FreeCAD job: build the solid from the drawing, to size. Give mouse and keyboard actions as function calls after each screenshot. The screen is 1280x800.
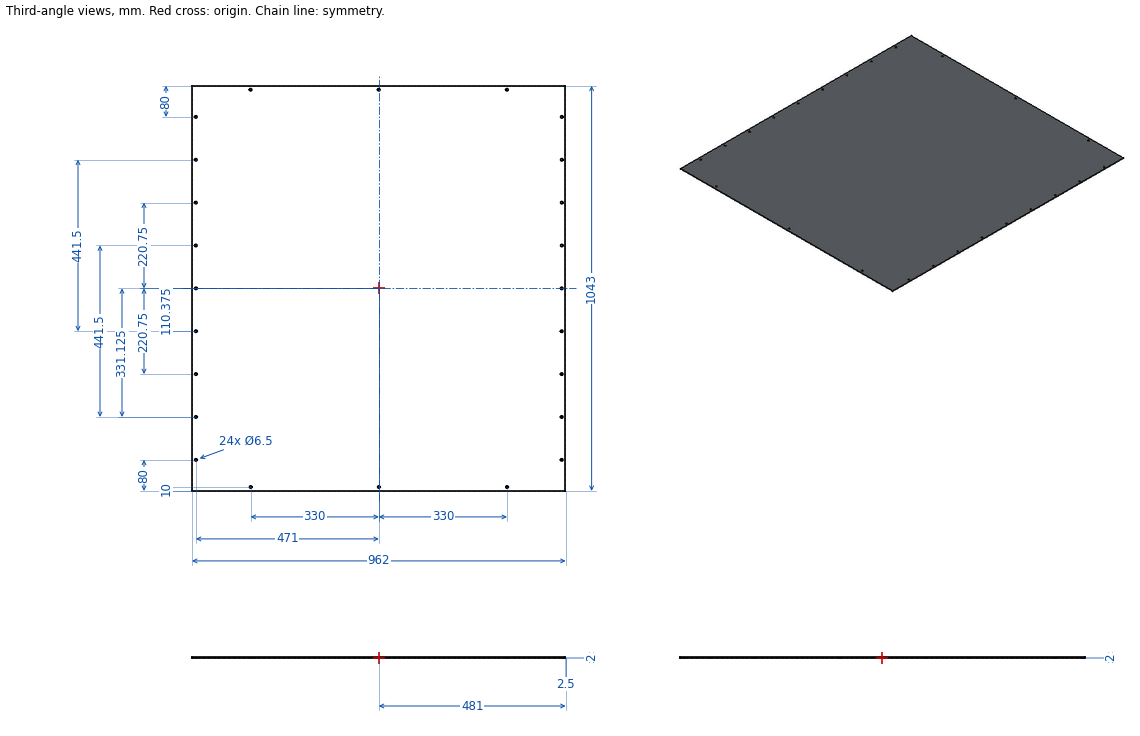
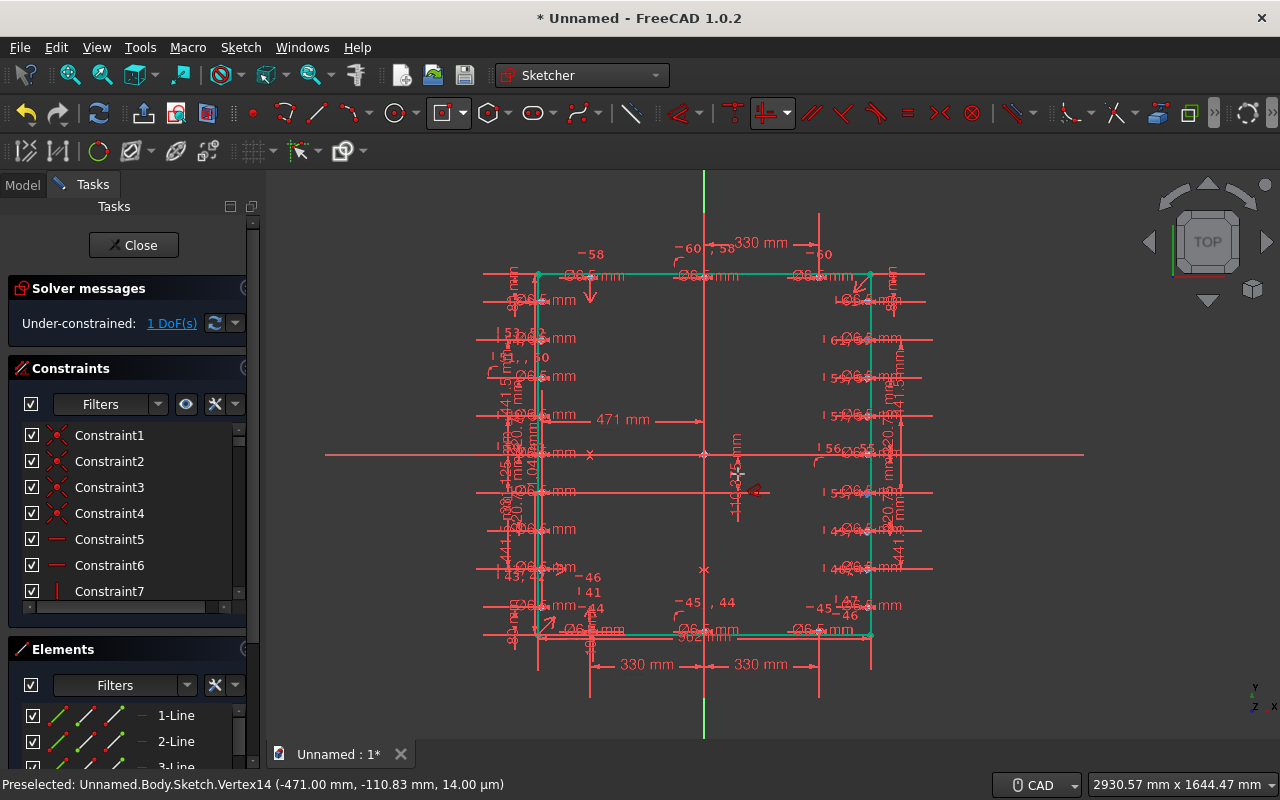
click(867, 493)
click(646, 474)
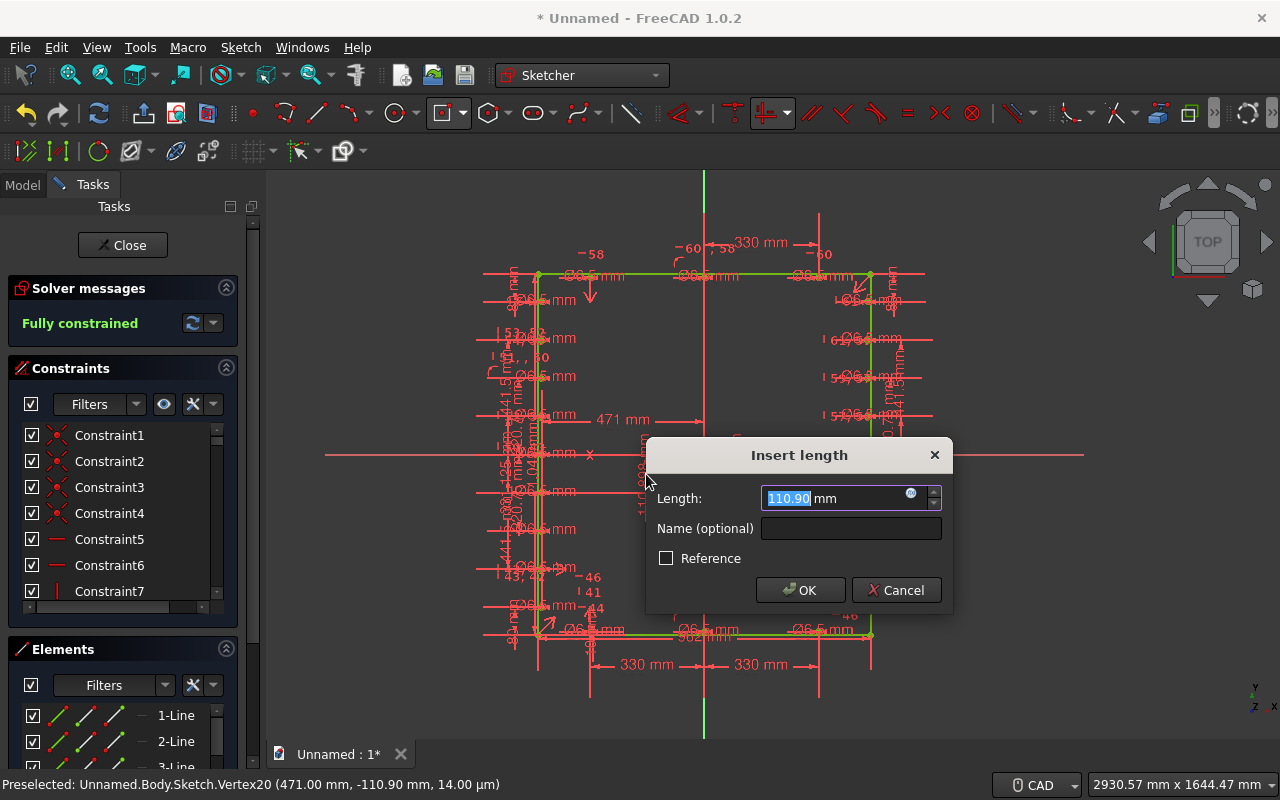
text(110.375)
key(Return)
key(Escape)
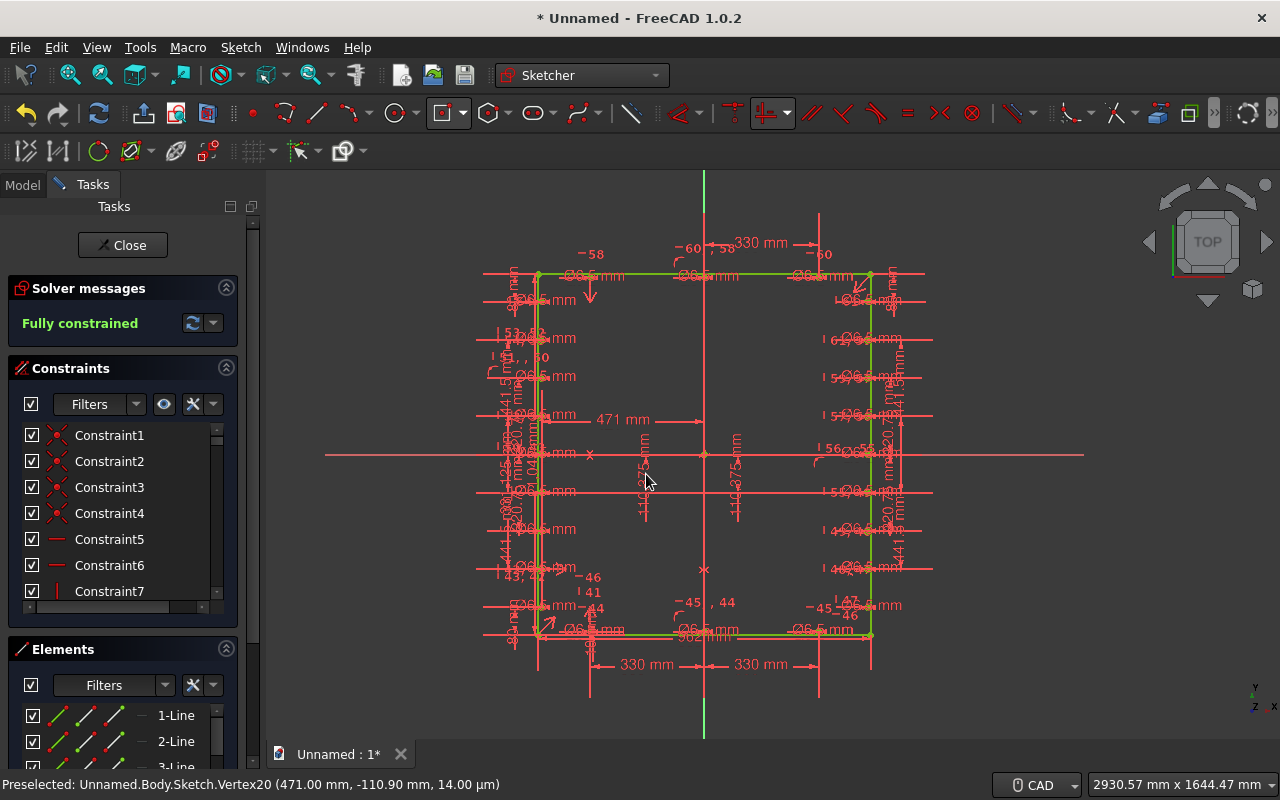
click(123, 245)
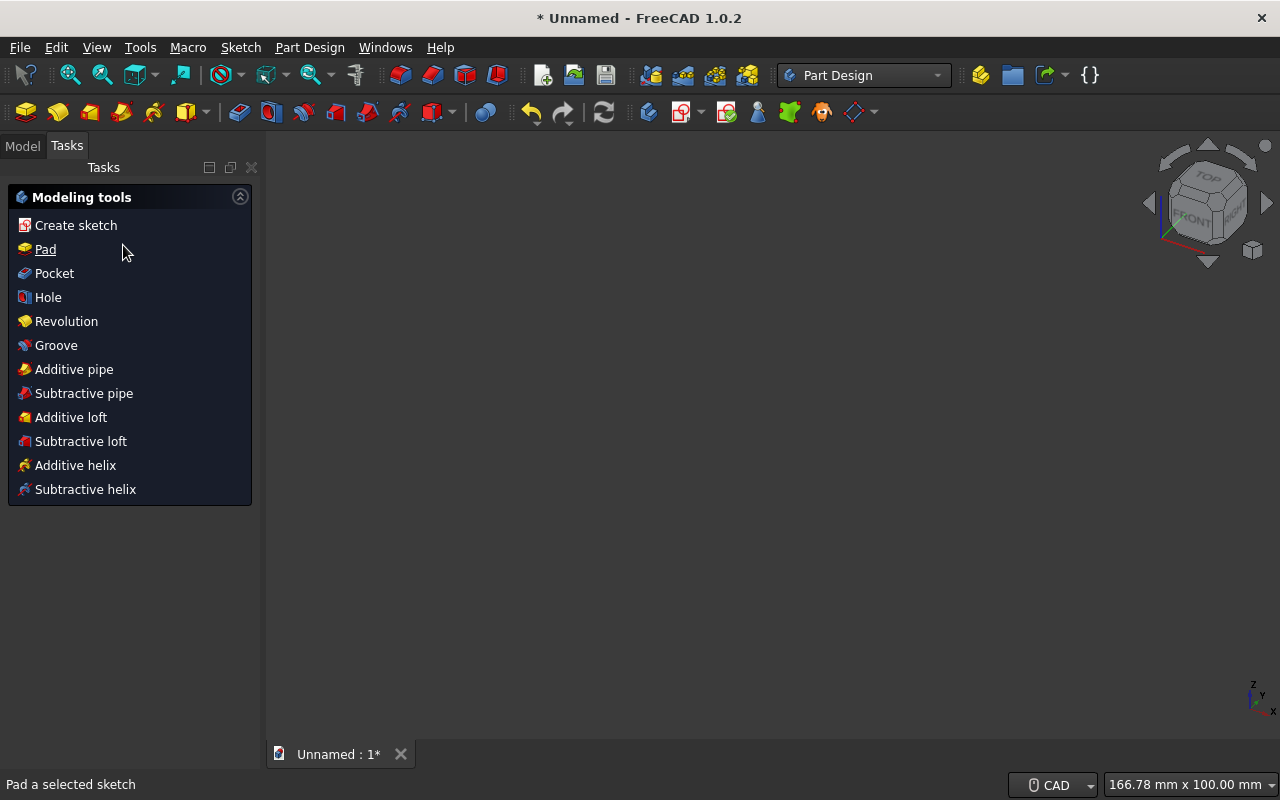
click(26, 112)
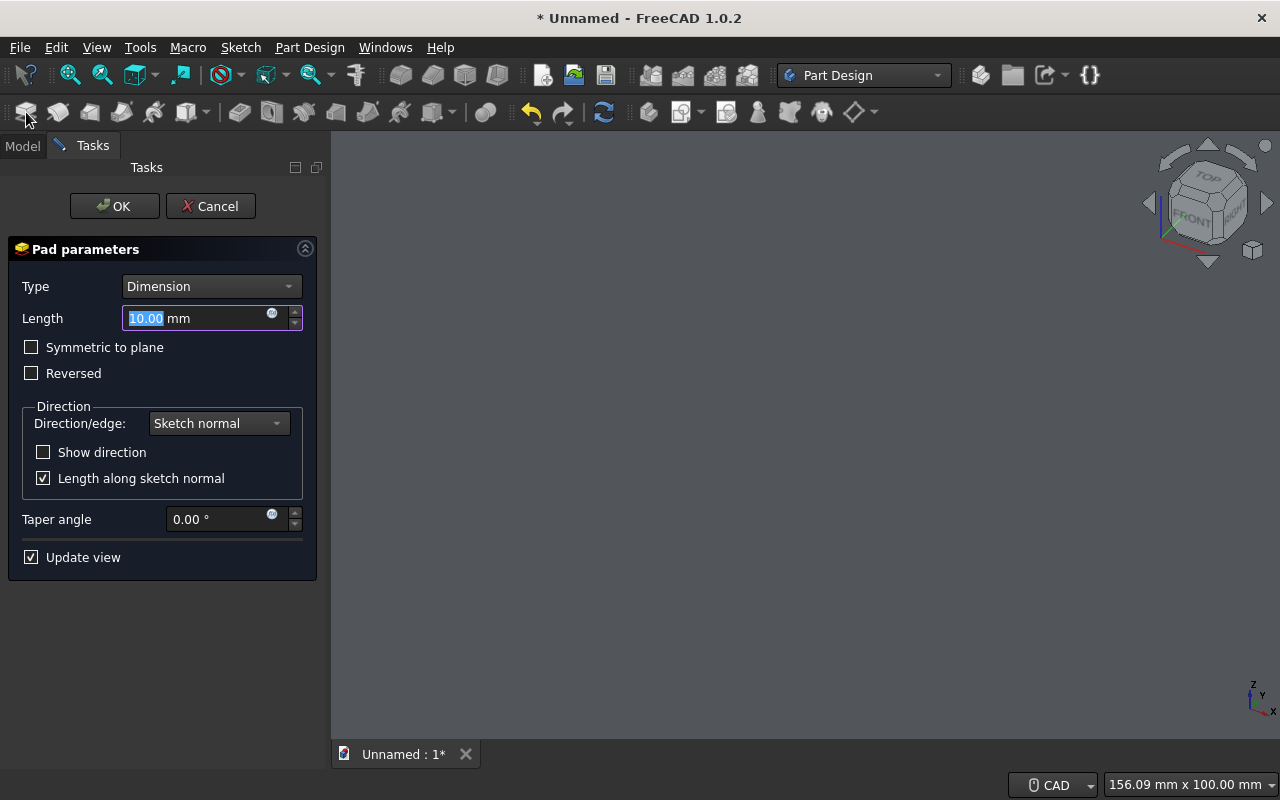
text(2)
key(Tab)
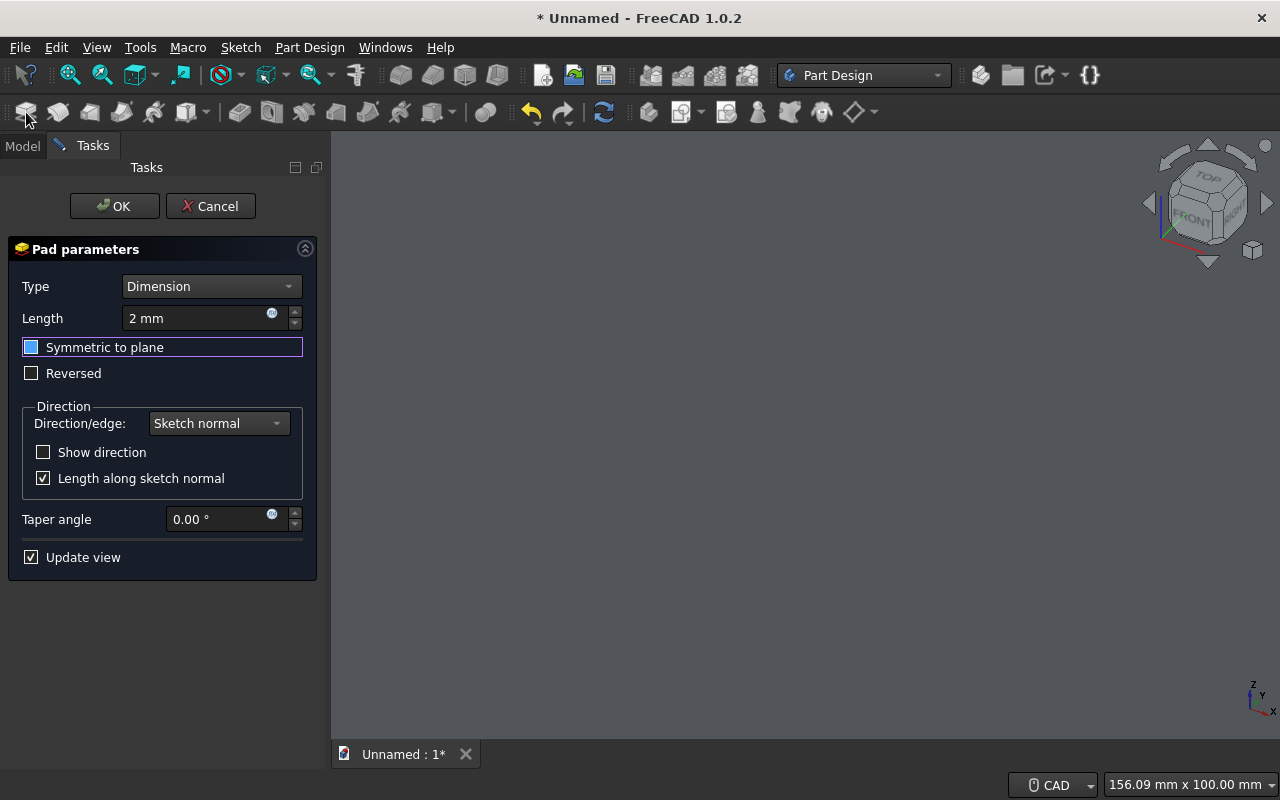
click(115, 206)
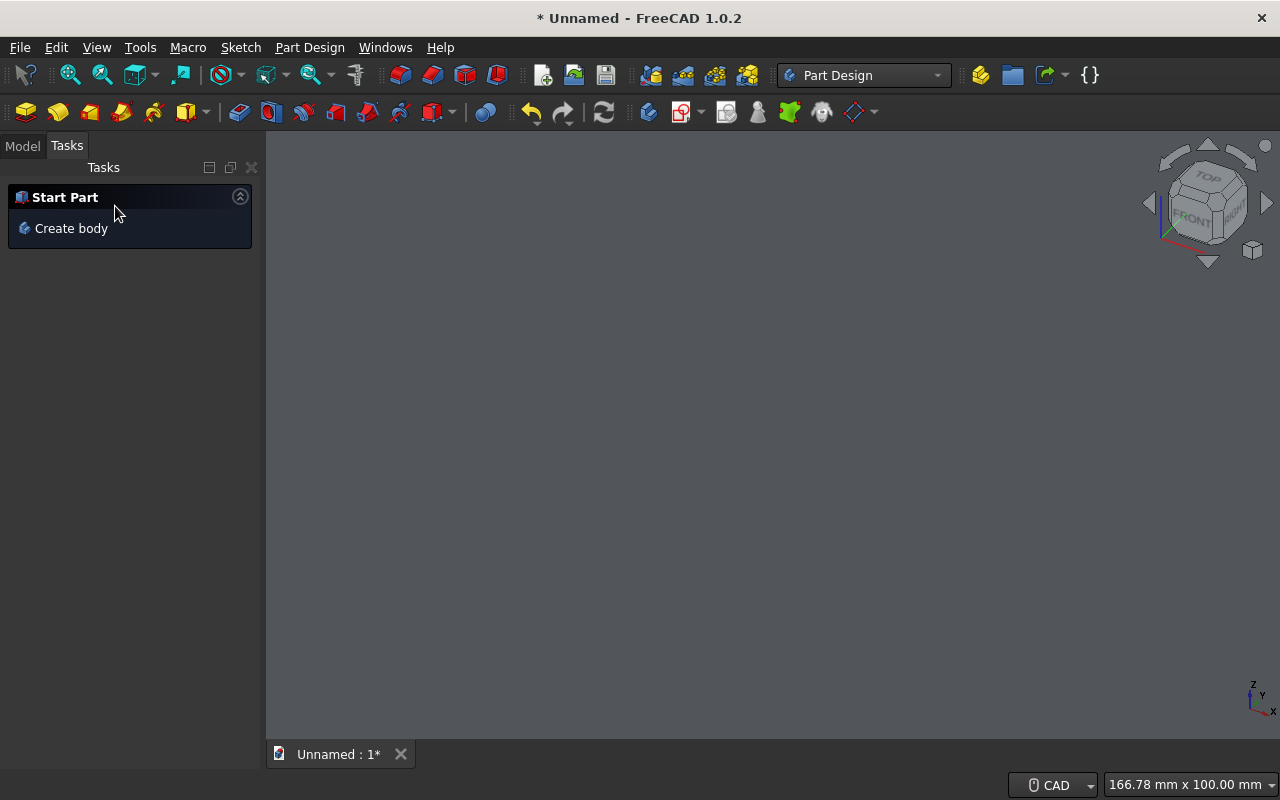
click(72, 76)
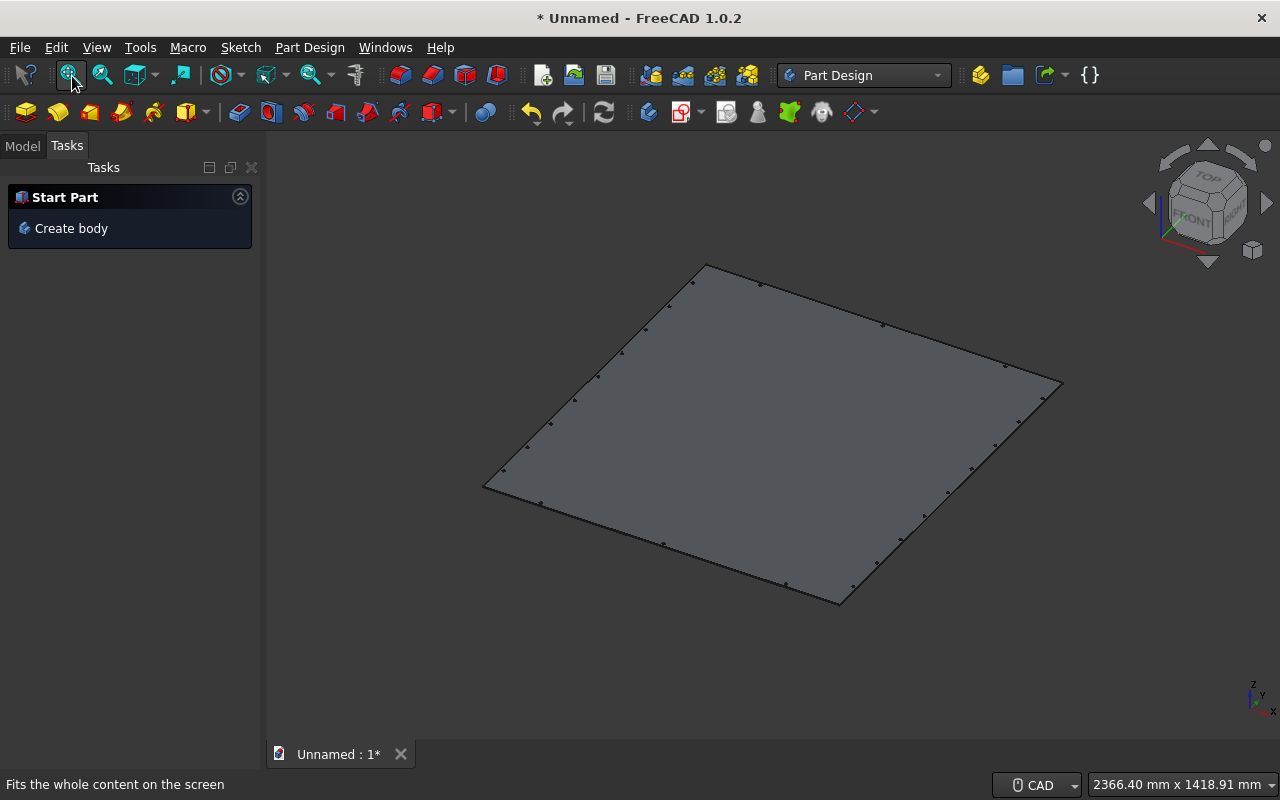
scroll(814, 596, up, 15)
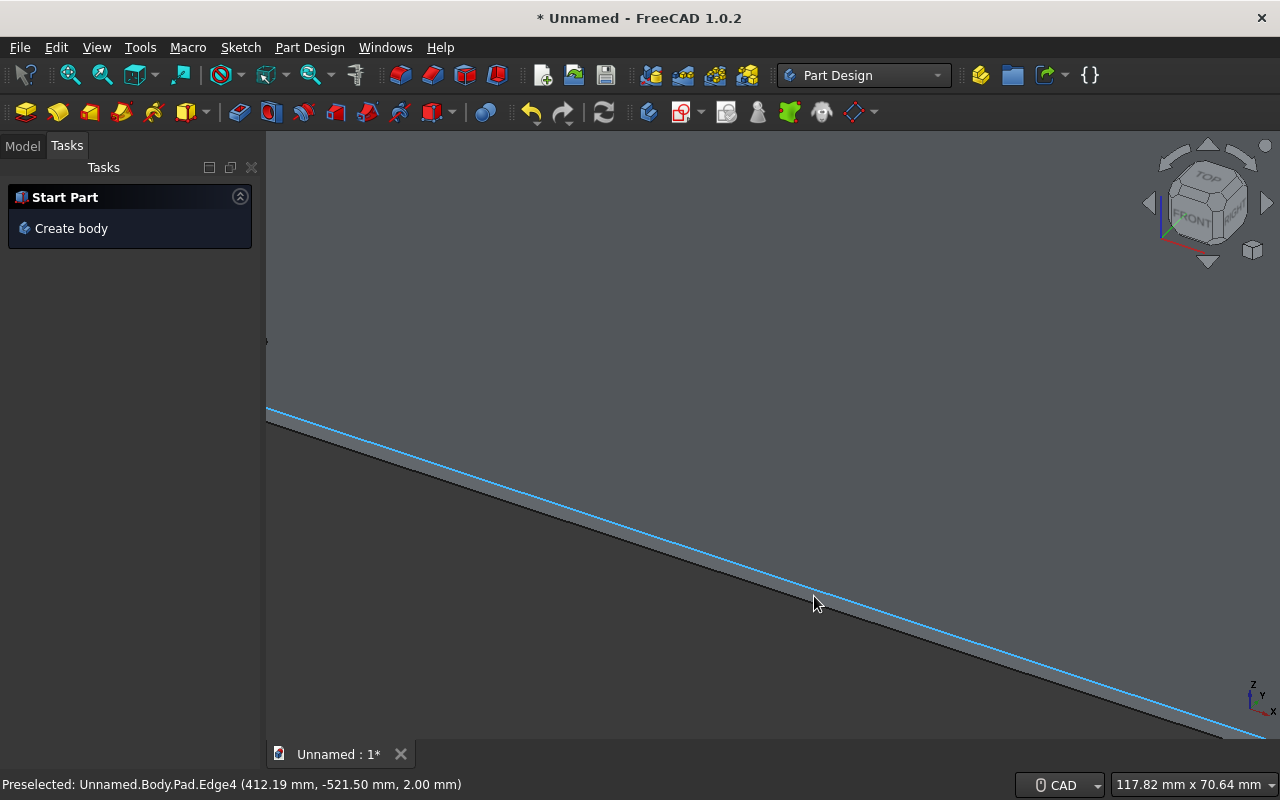
click(72, 76)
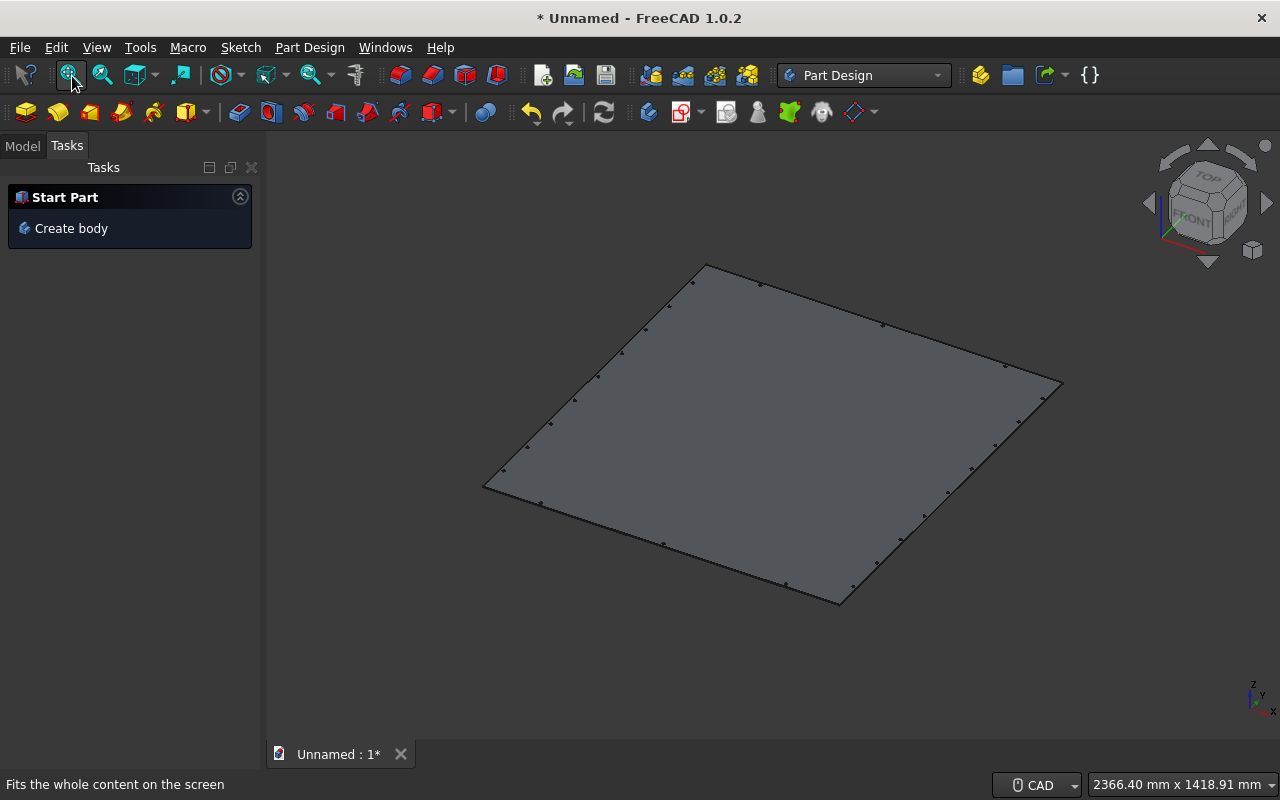
key(0)